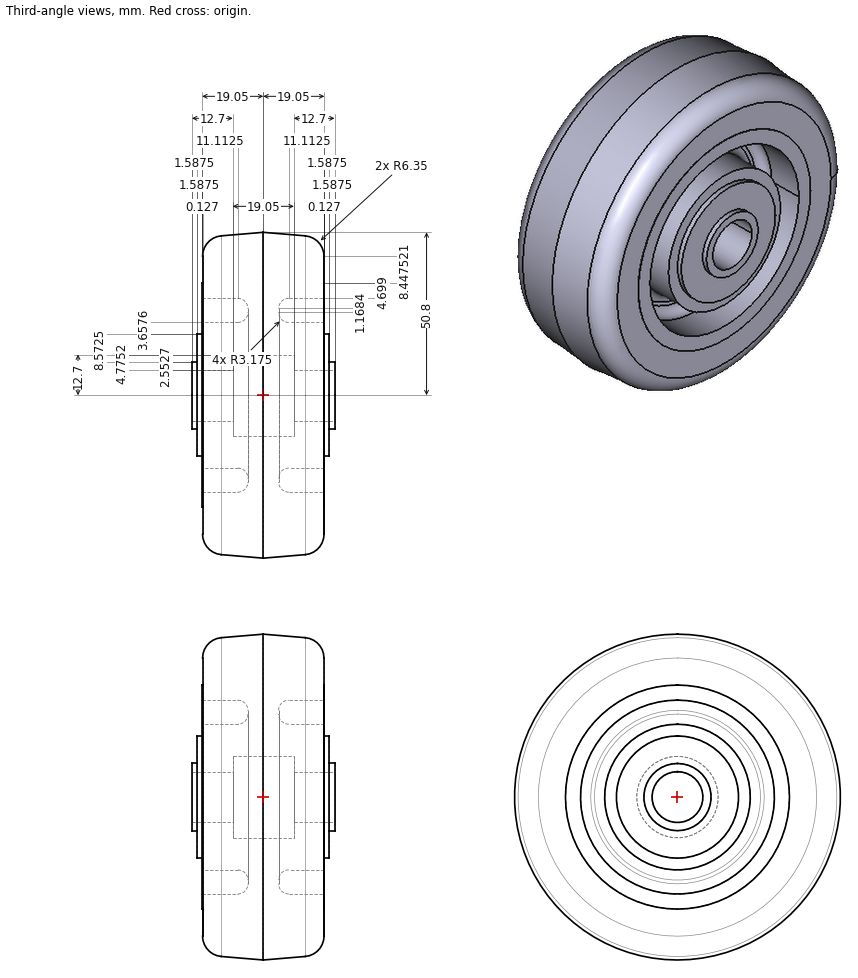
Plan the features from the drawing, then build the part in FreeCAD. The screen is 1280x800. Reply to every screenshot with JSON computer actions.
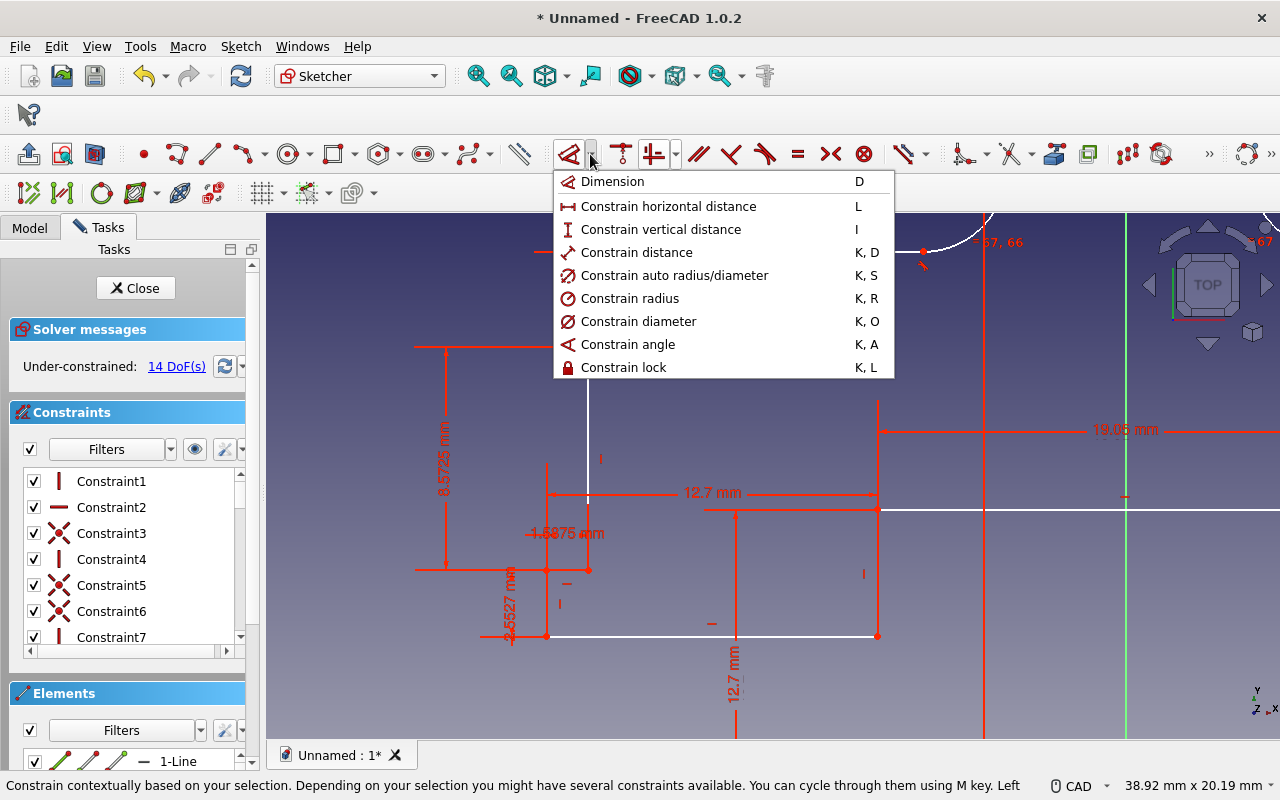
{"action": "left_click", "coordinate": [724, 230]}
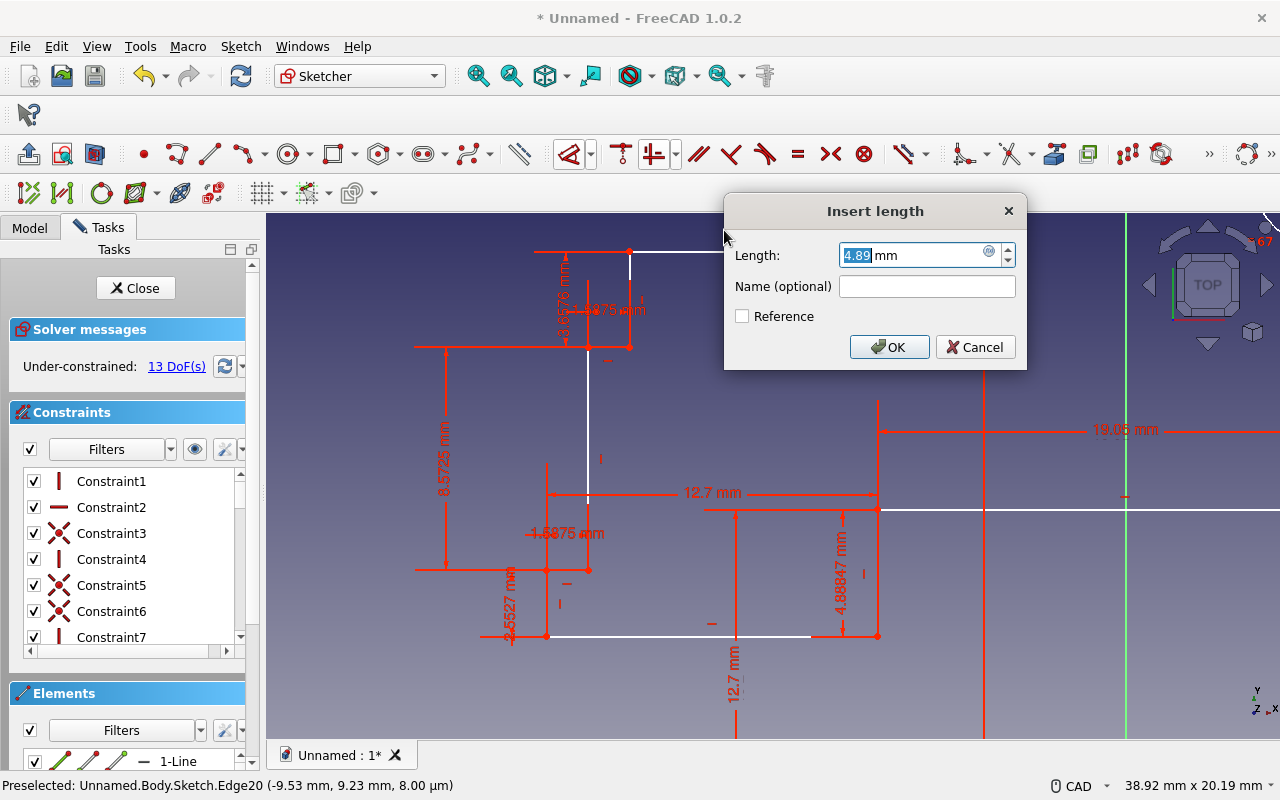
{"action": "type", "text": "4.7752"}
{"action": "key", "text": "Return"}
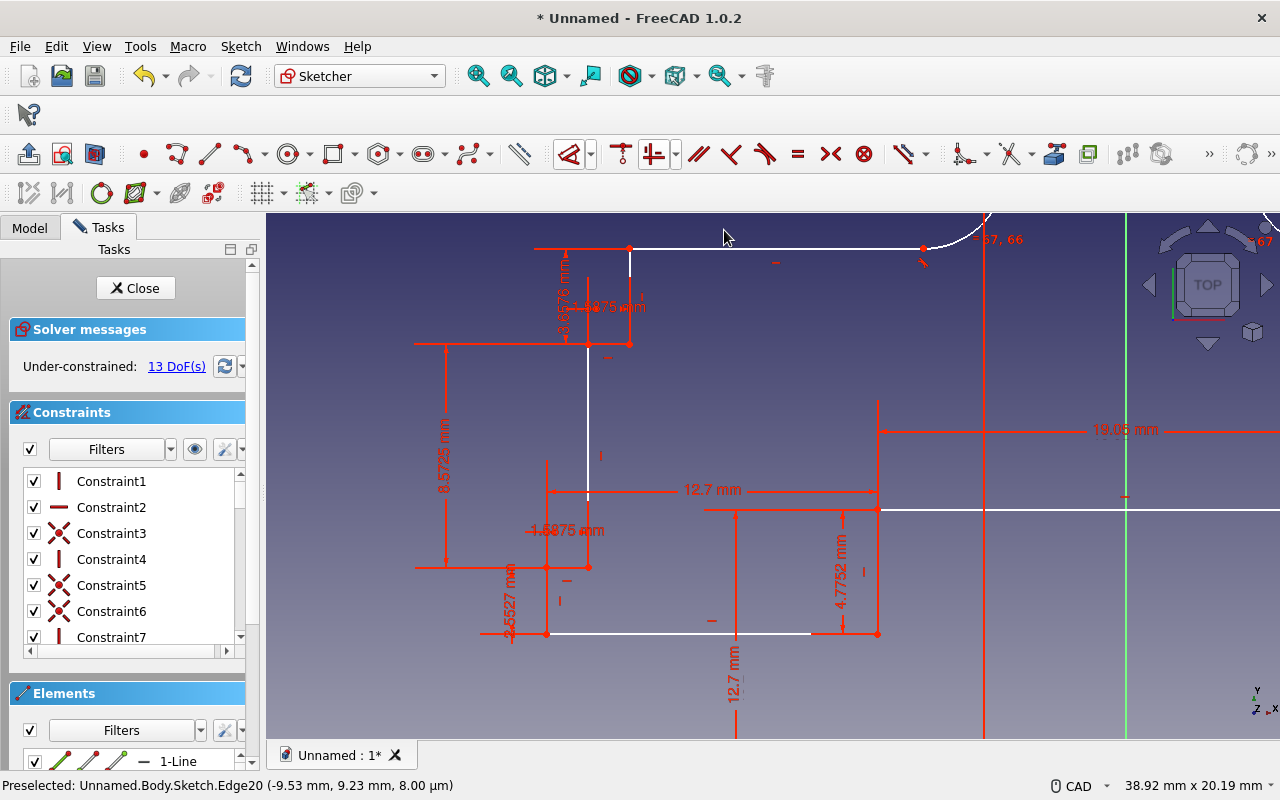
{"action": "scroll", "coordinate": [567, 573], "scroll_direction": "down", "scroll_amount": 7}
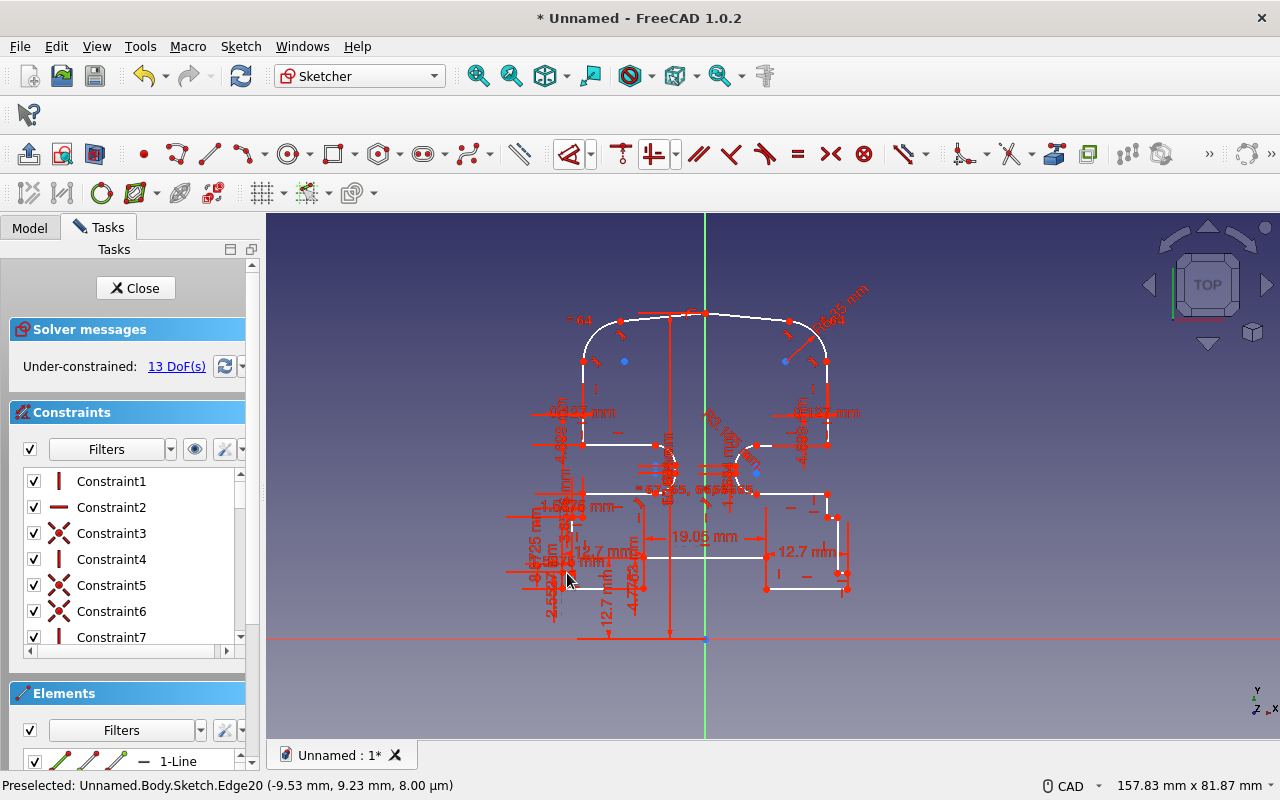
{"action": "scroll", "coordinate": [766, 567], "scroll_direction": "up", "scroll_amount": 2}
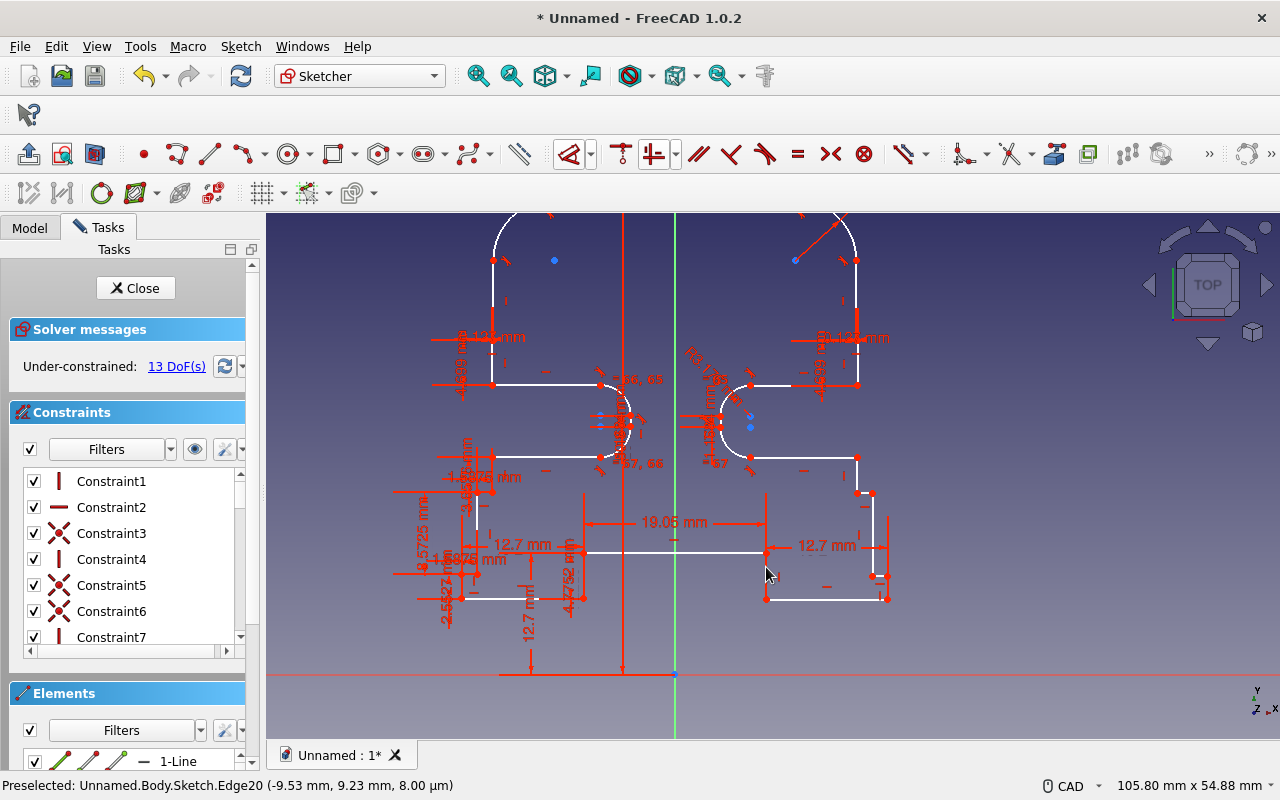
{"action": "left_click", "coordinate": [766, 567]}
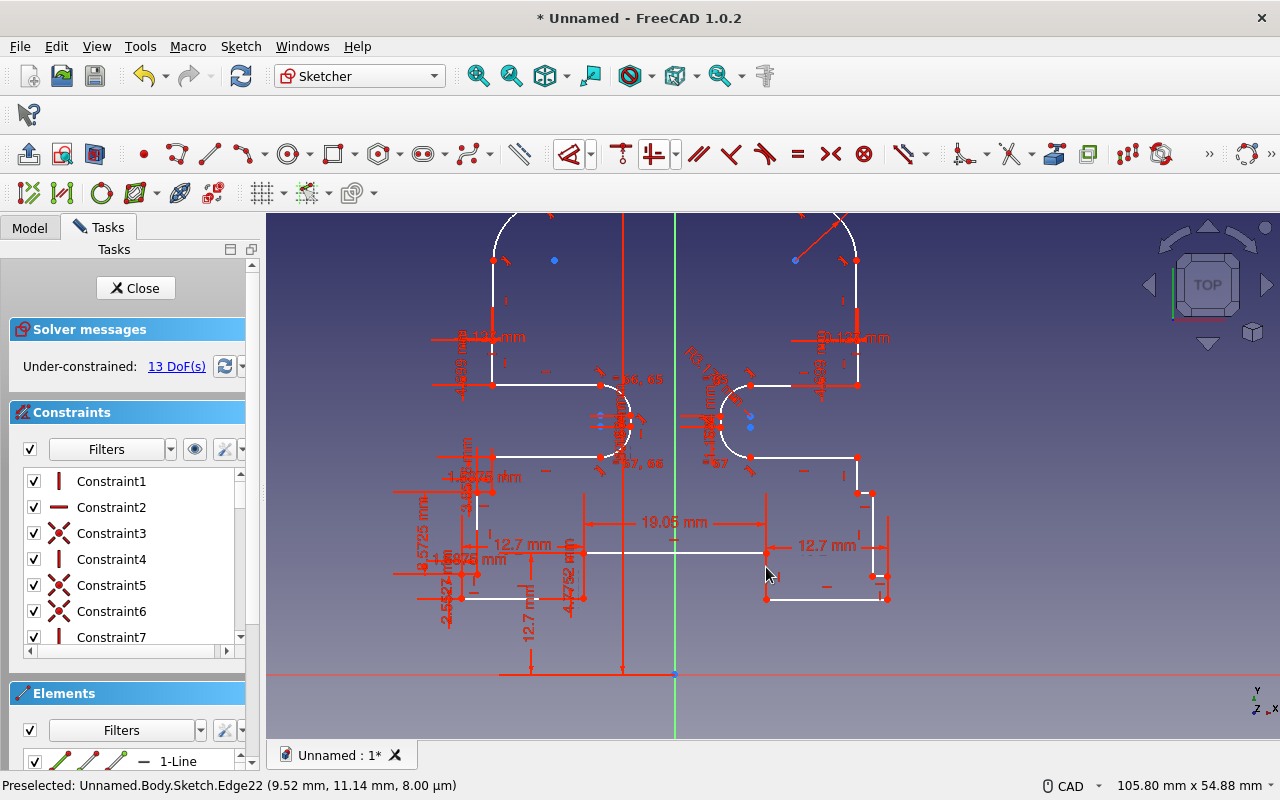
{"action": "left_click", "coordinate": [590, 154]}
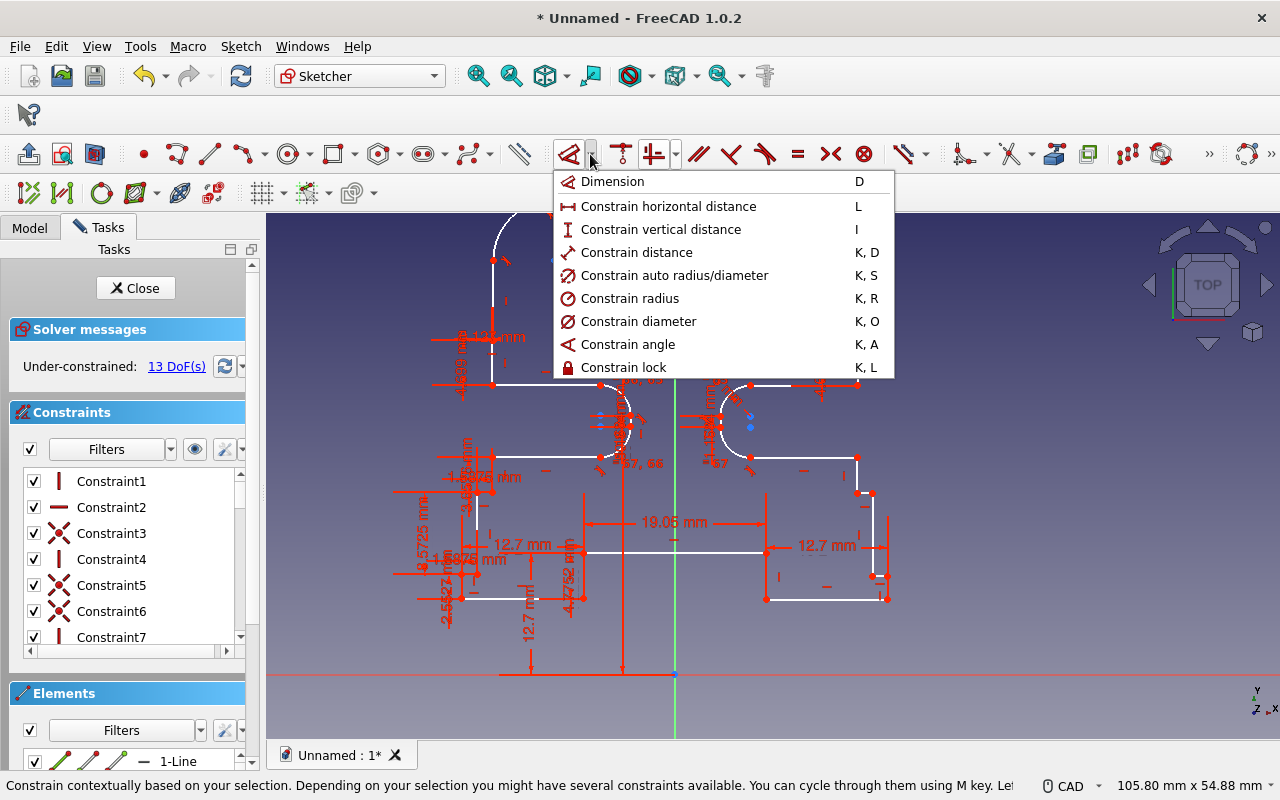
{"action": "left_click", "coordinate": [724, 230]}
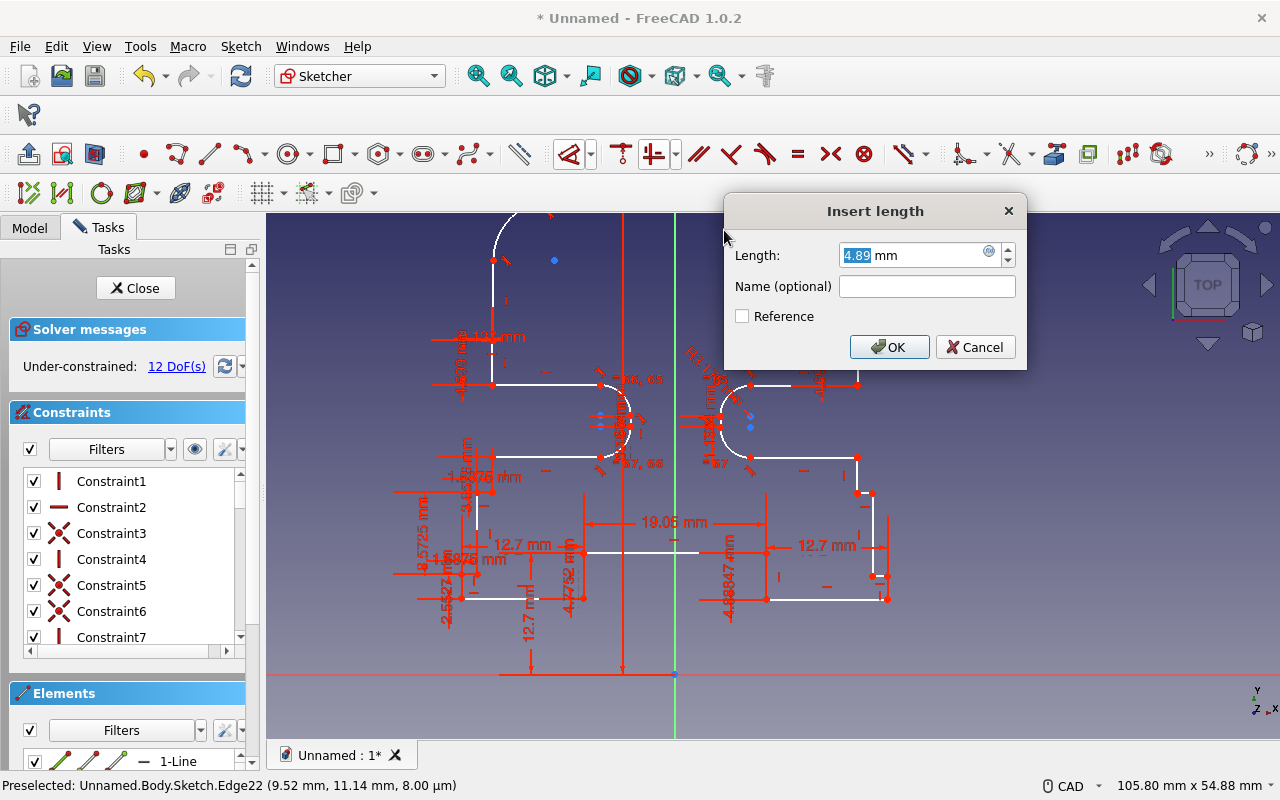
{"action": "type", "text": "4.7752"}
{"action": "key", "text": "Return"}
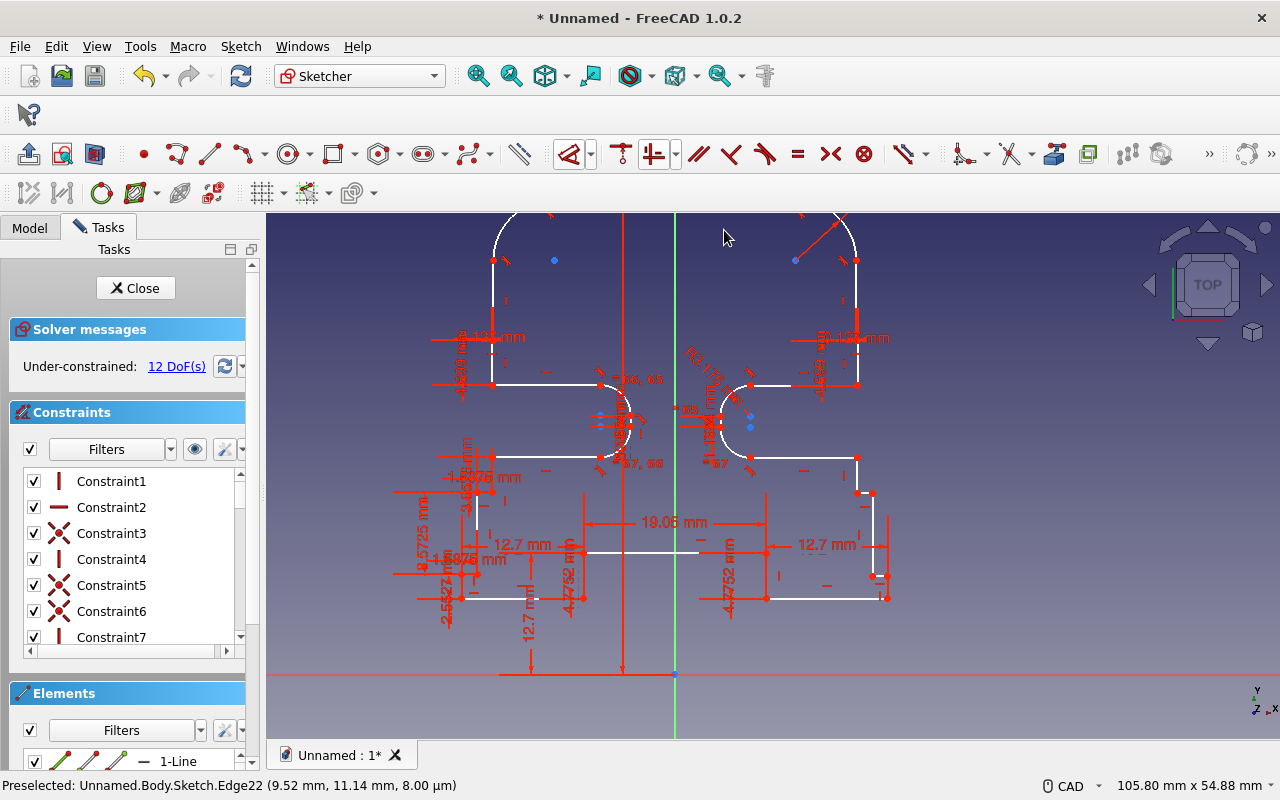
{"action": "scroll", "coordinate": [888, 590], "scroll_direction": "up", "scroll_amount": 3}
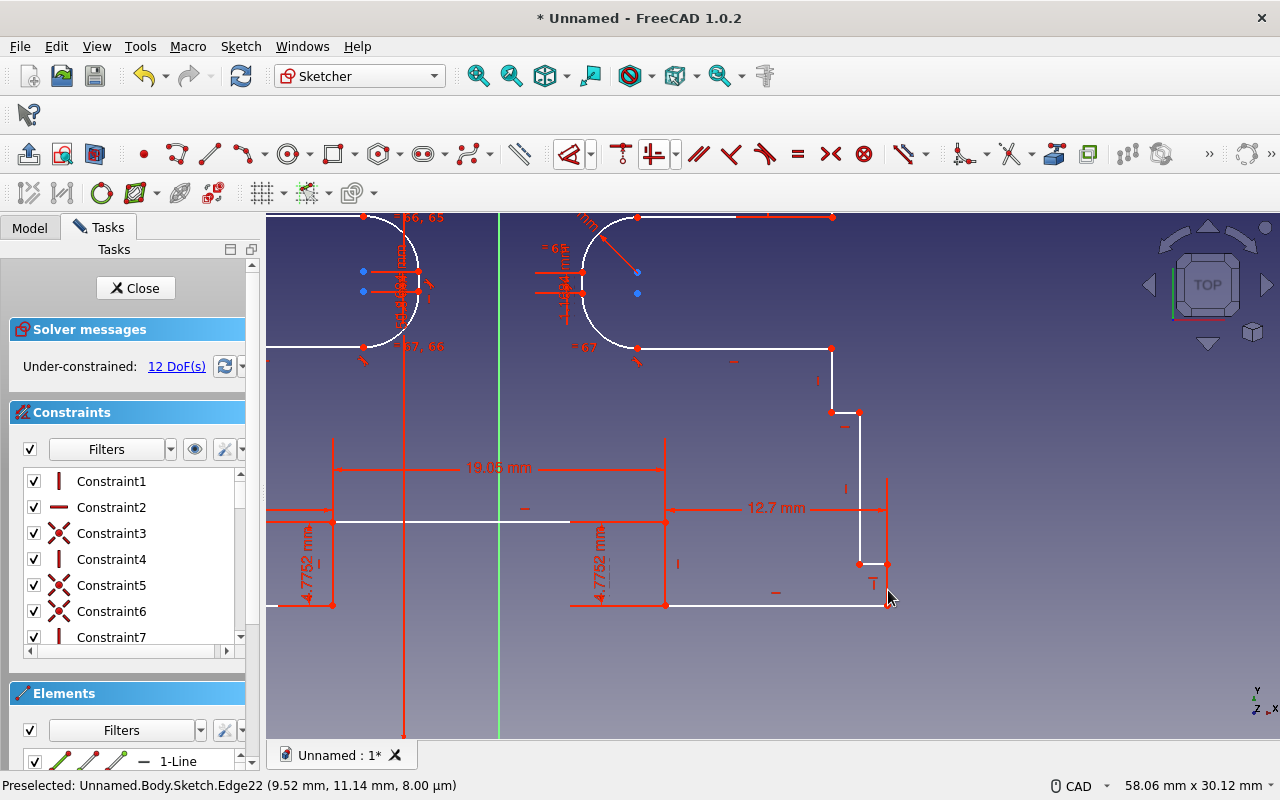
{"action": "left_click", "coordinate": [887, 589]}